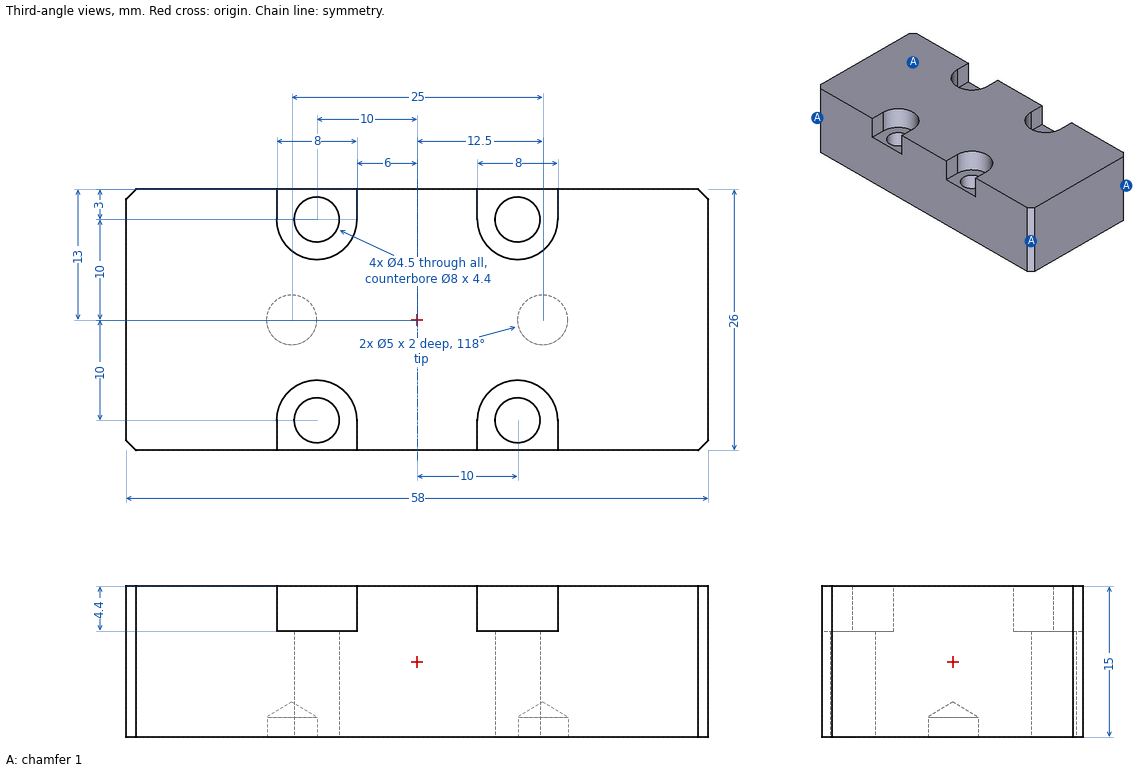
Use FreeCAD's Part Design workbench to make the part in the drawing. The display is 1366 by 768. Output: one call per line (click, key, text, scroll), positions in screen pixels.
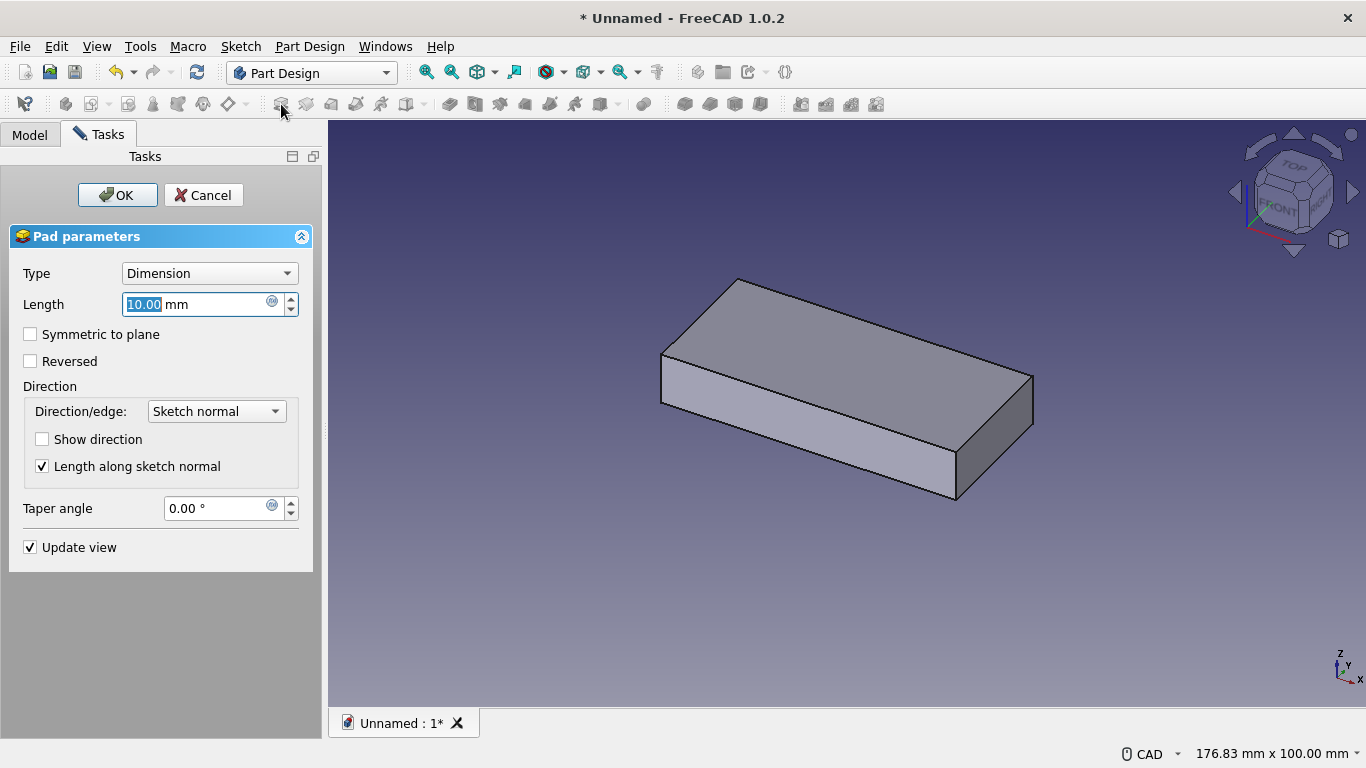
text(15)
key(Tab)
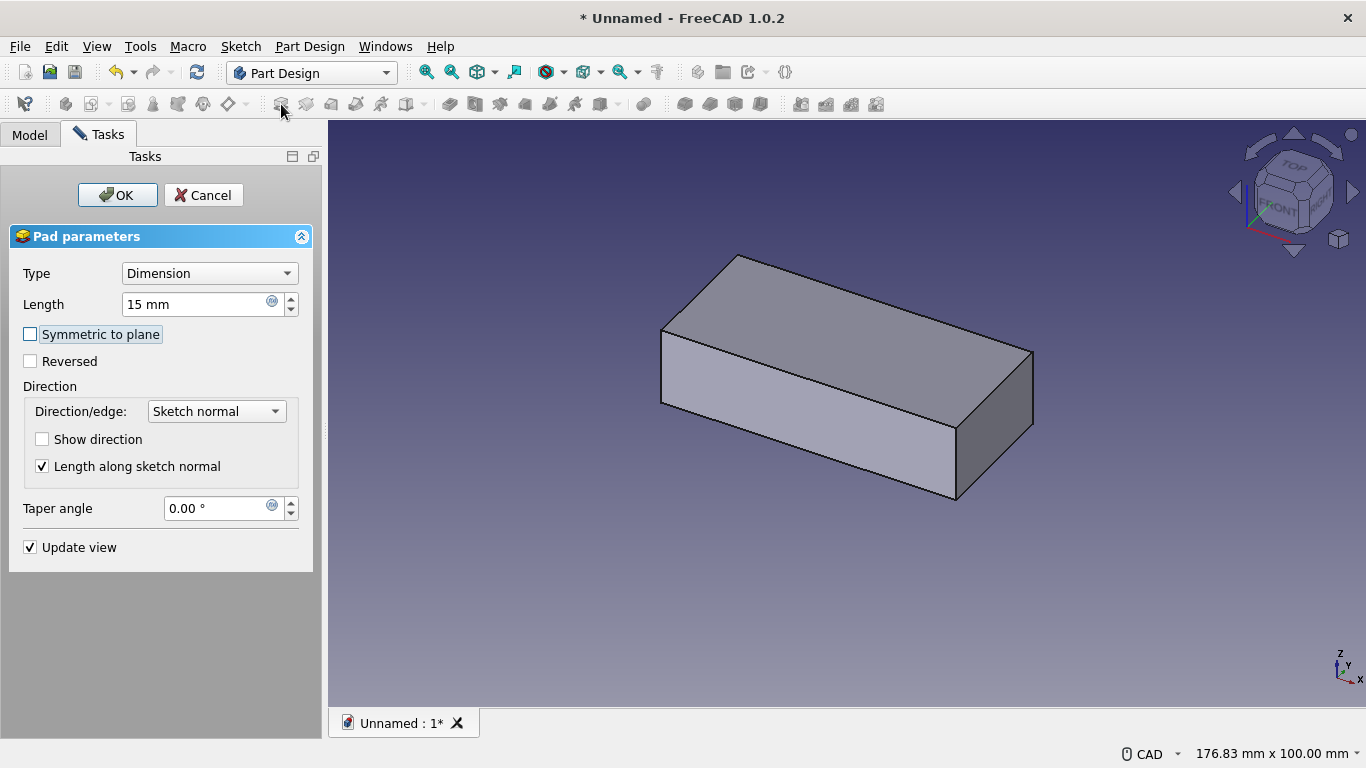
click(31, 334)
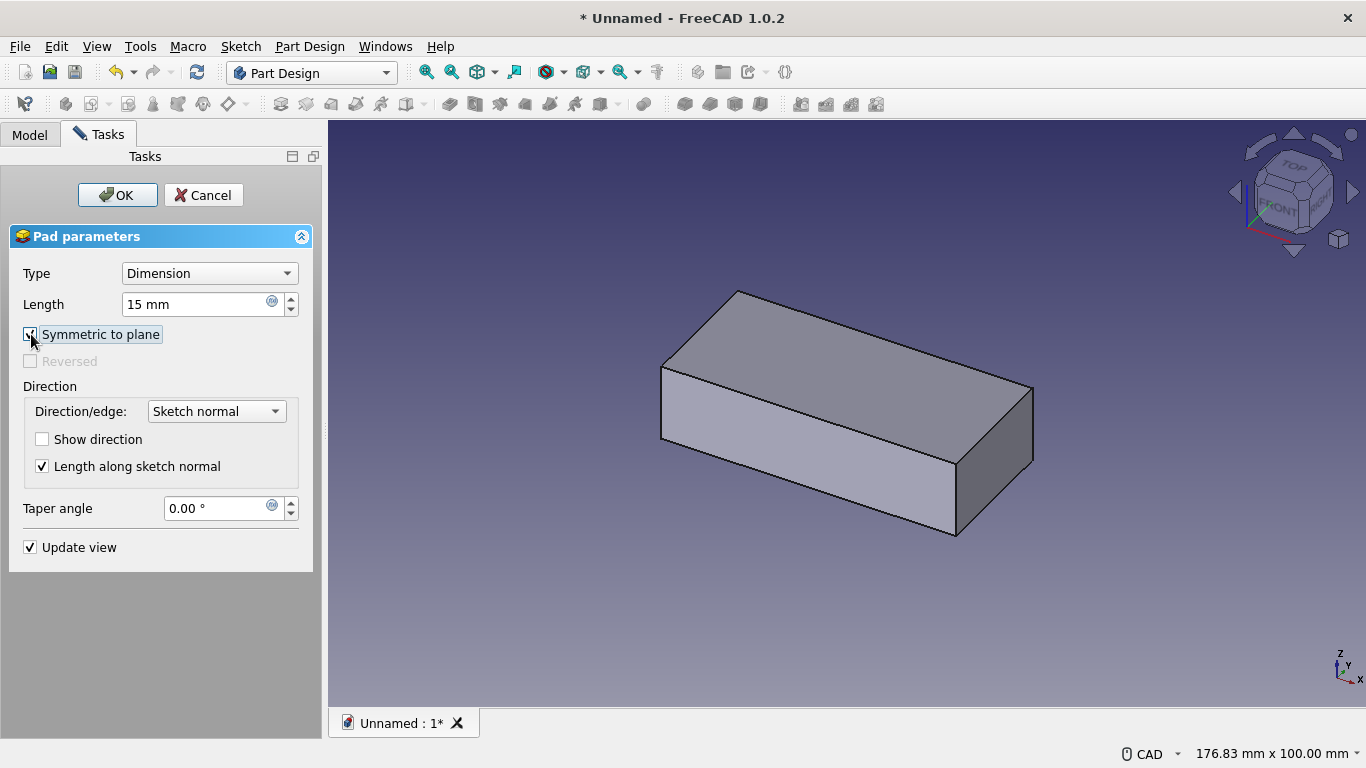
click(118, 195)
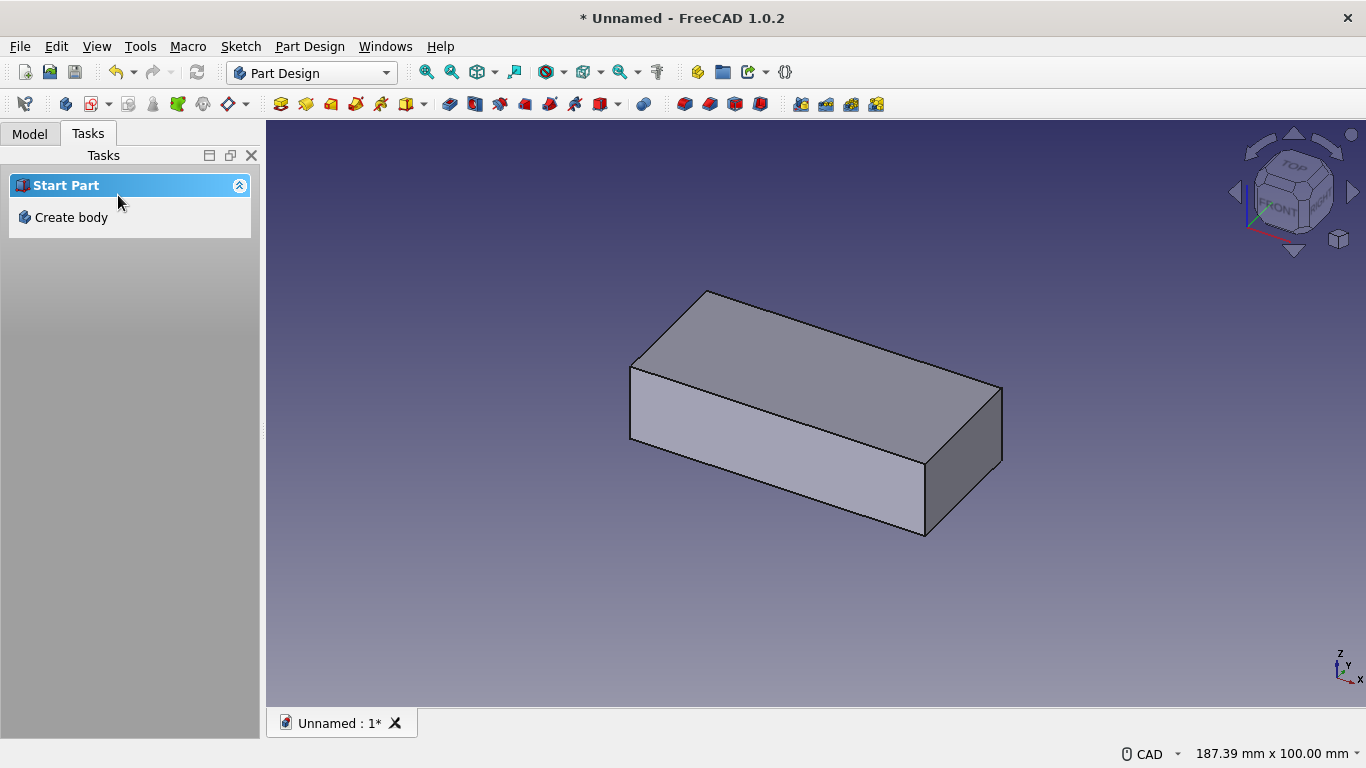
key(v)
key(f)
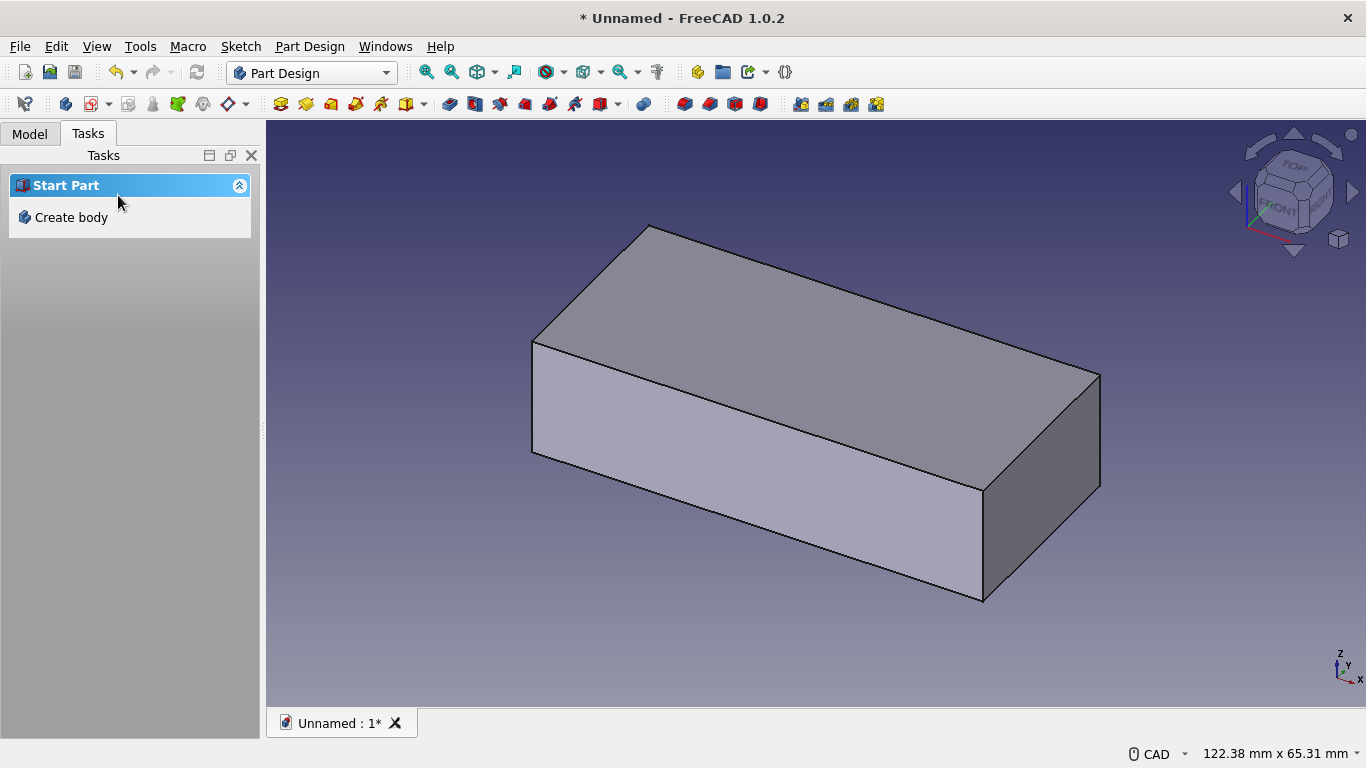
click(880, 379)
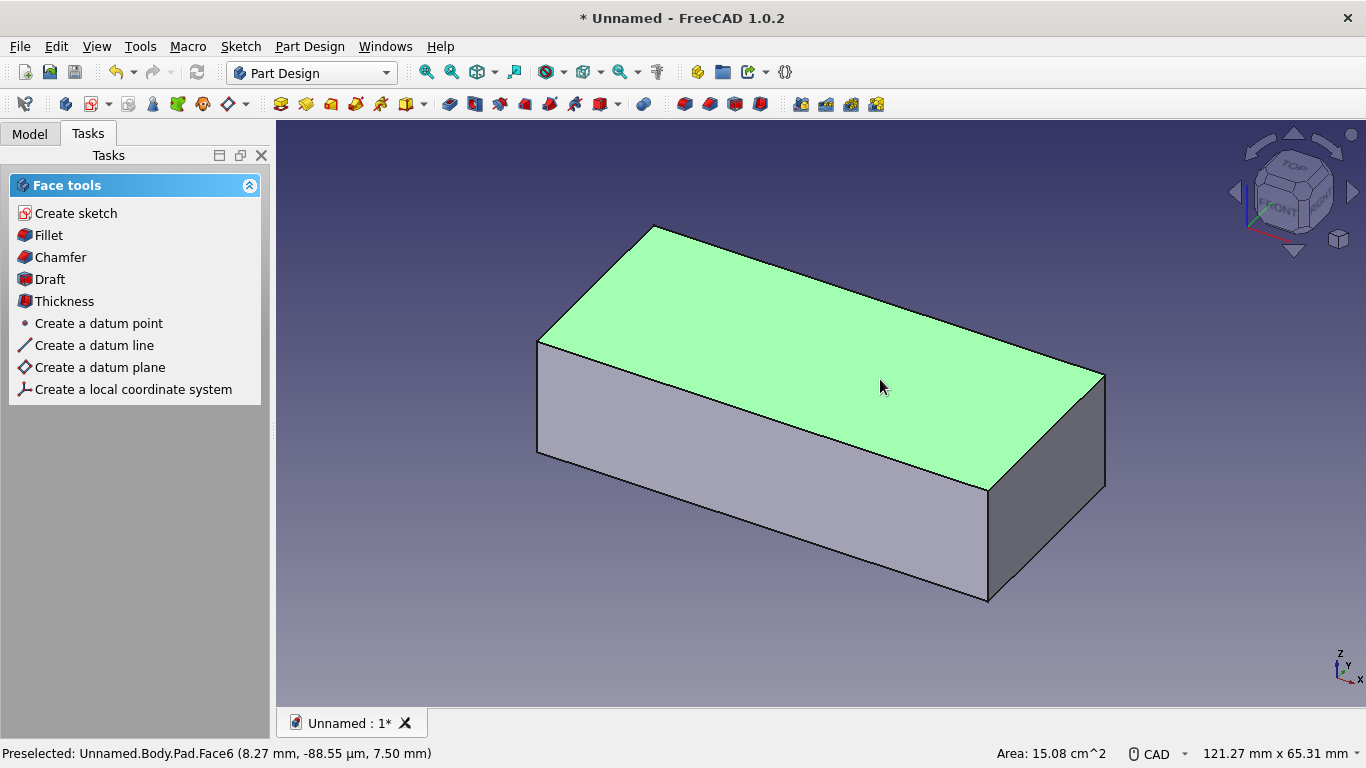
click(90, 104)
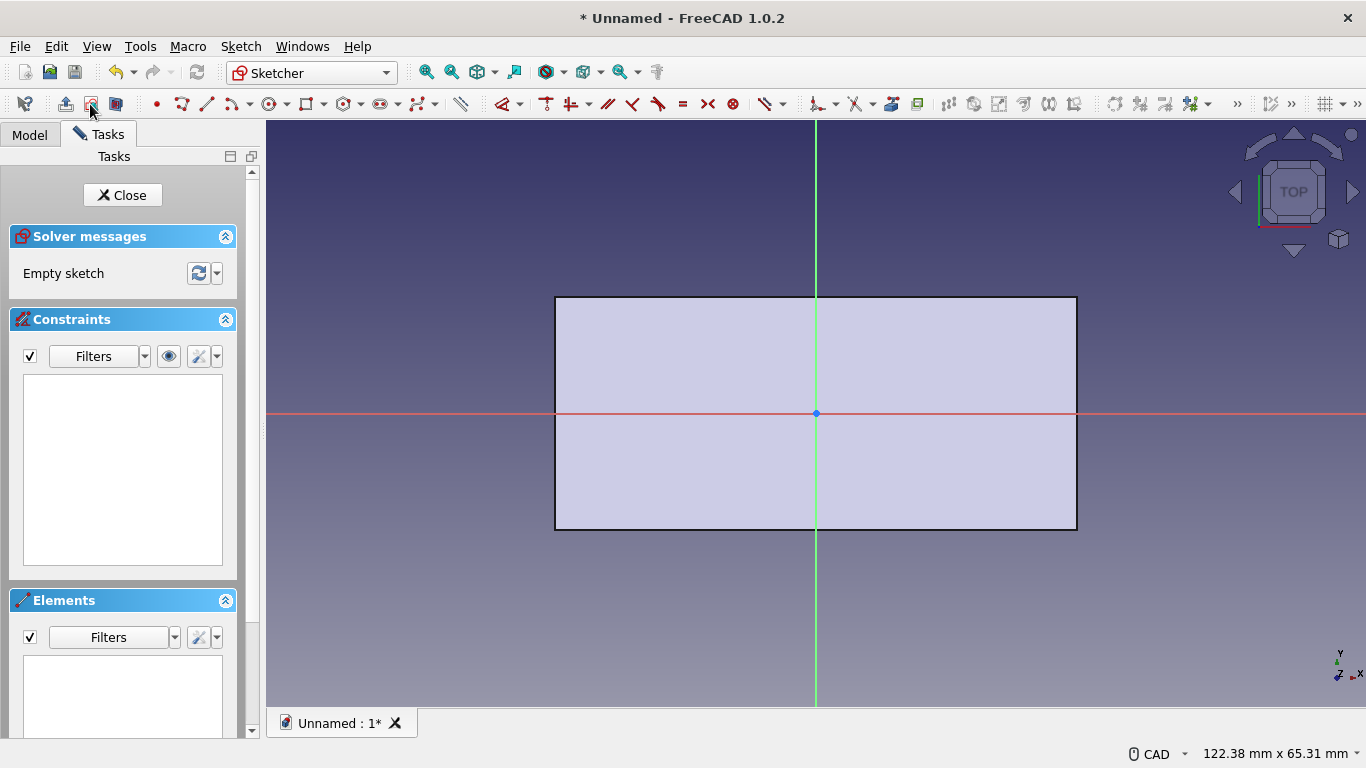
scroll(899, 414, up, 3)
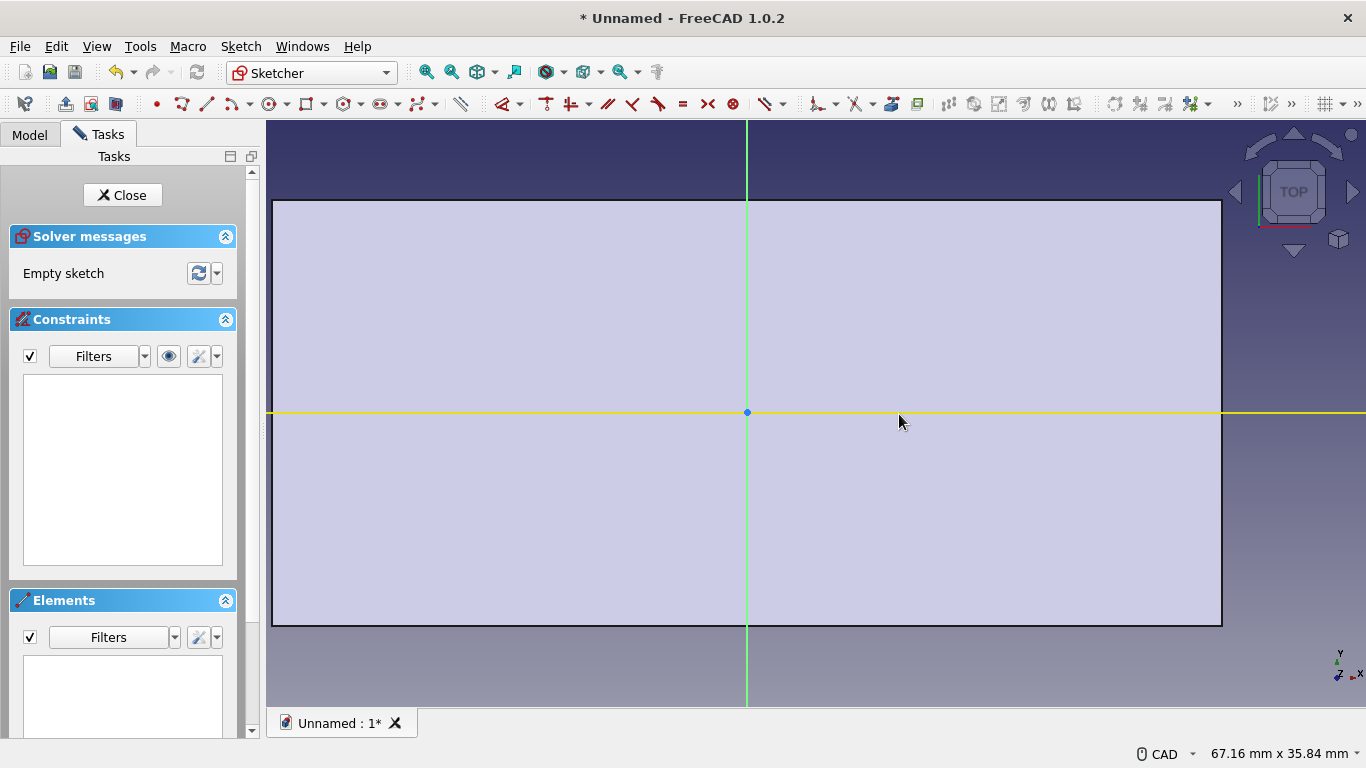
key(g)
key(c)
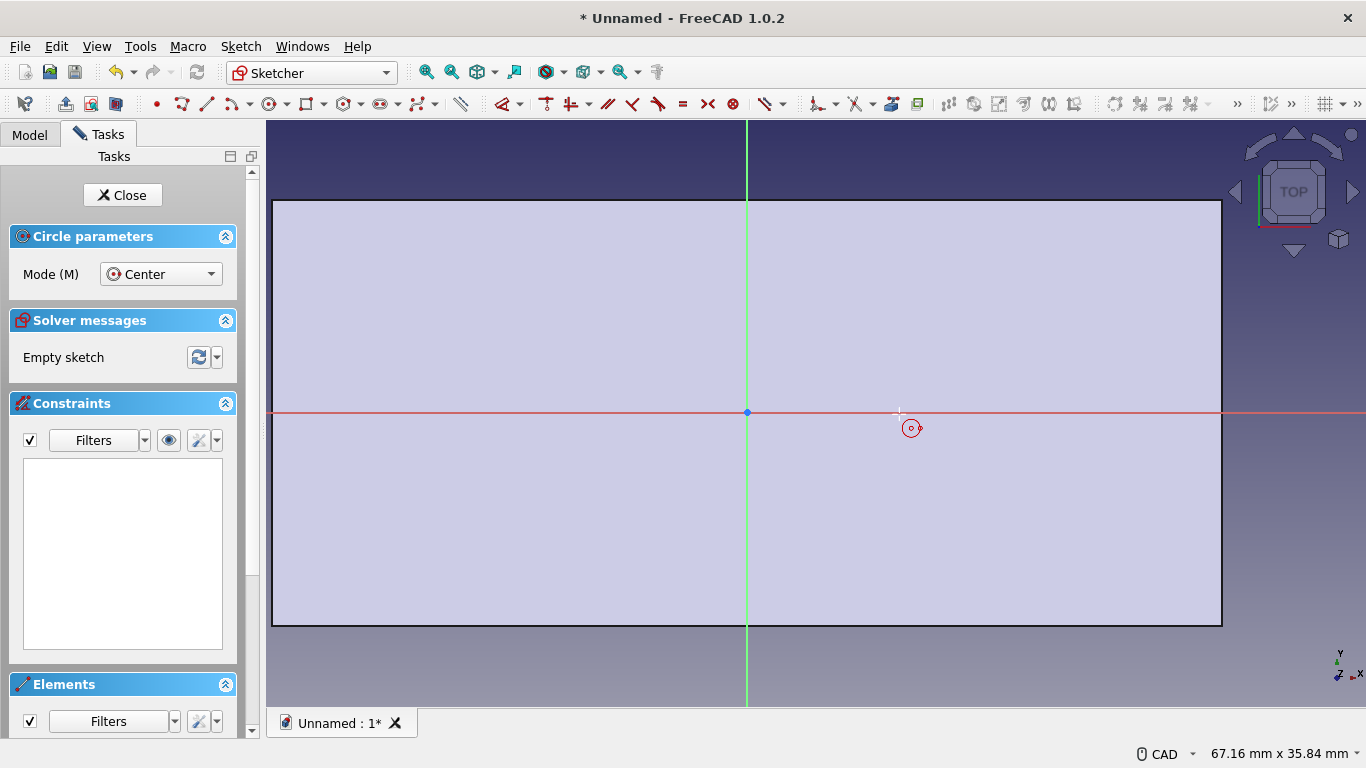
click(584, 249)
move(610, 223)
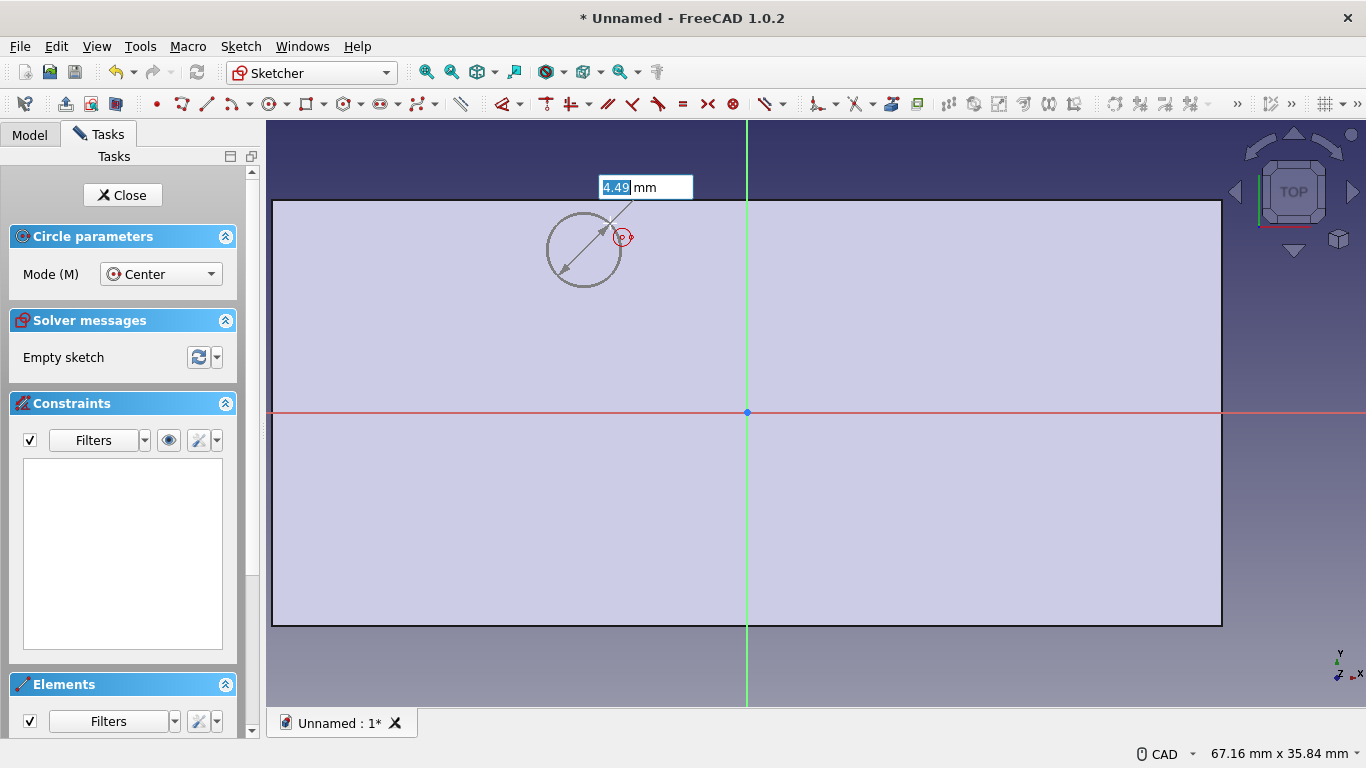
text(4.5)
key(Return)